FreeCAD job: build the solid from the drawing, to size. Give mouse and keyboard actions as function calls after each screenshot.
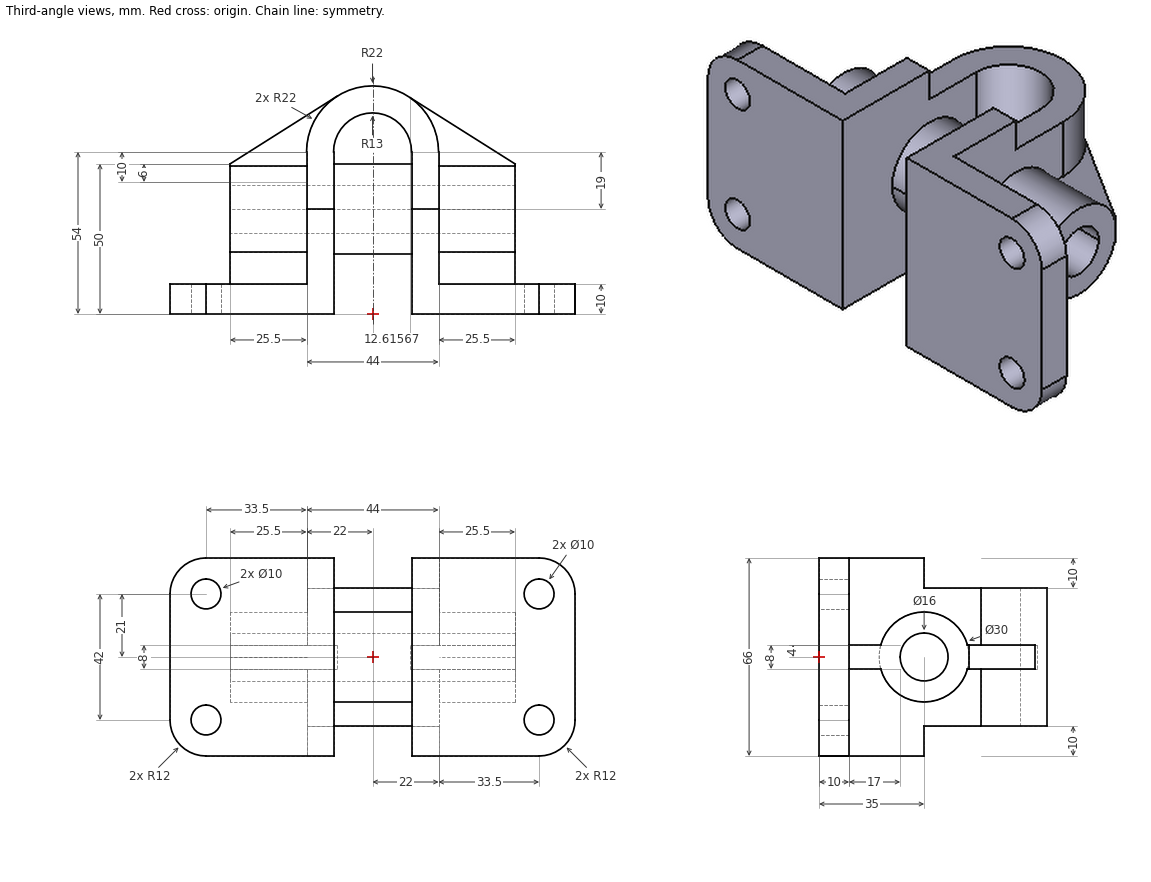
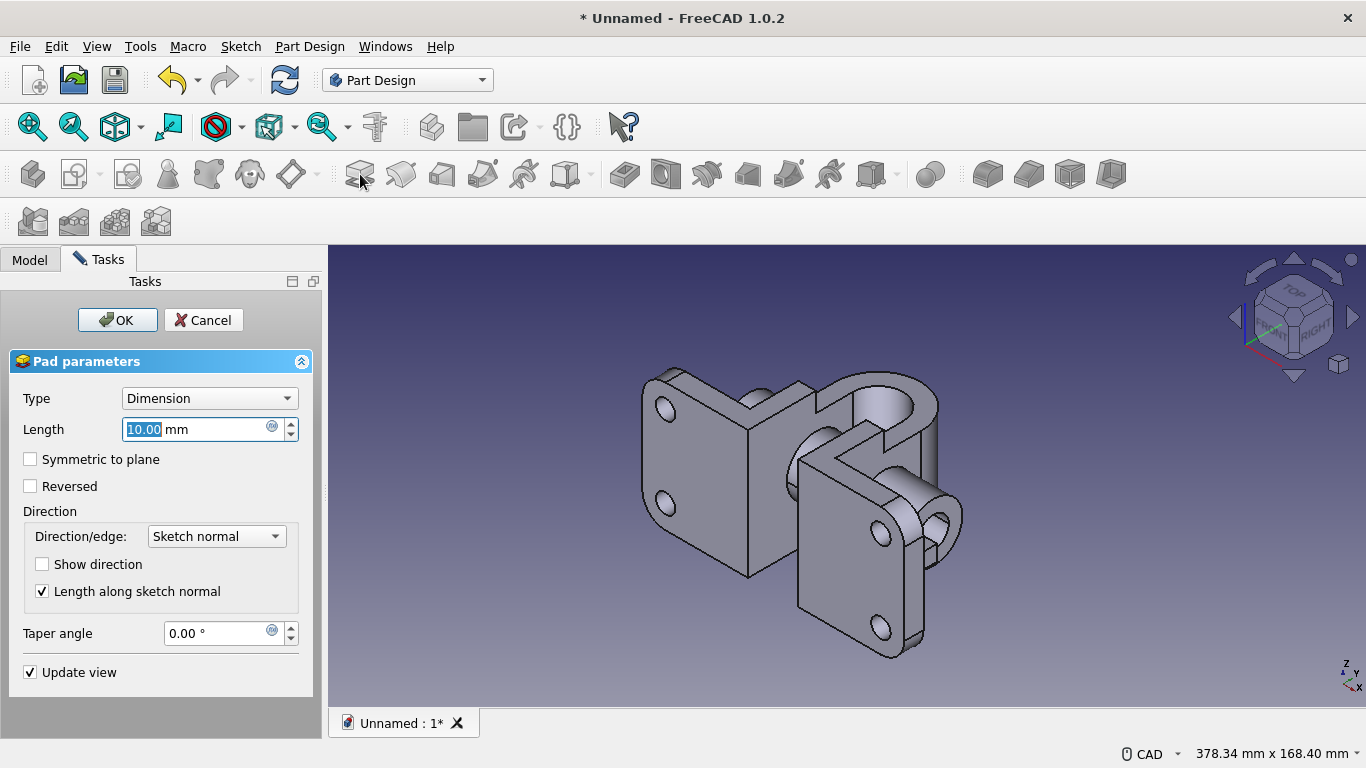
text(25.5)
key(Tab)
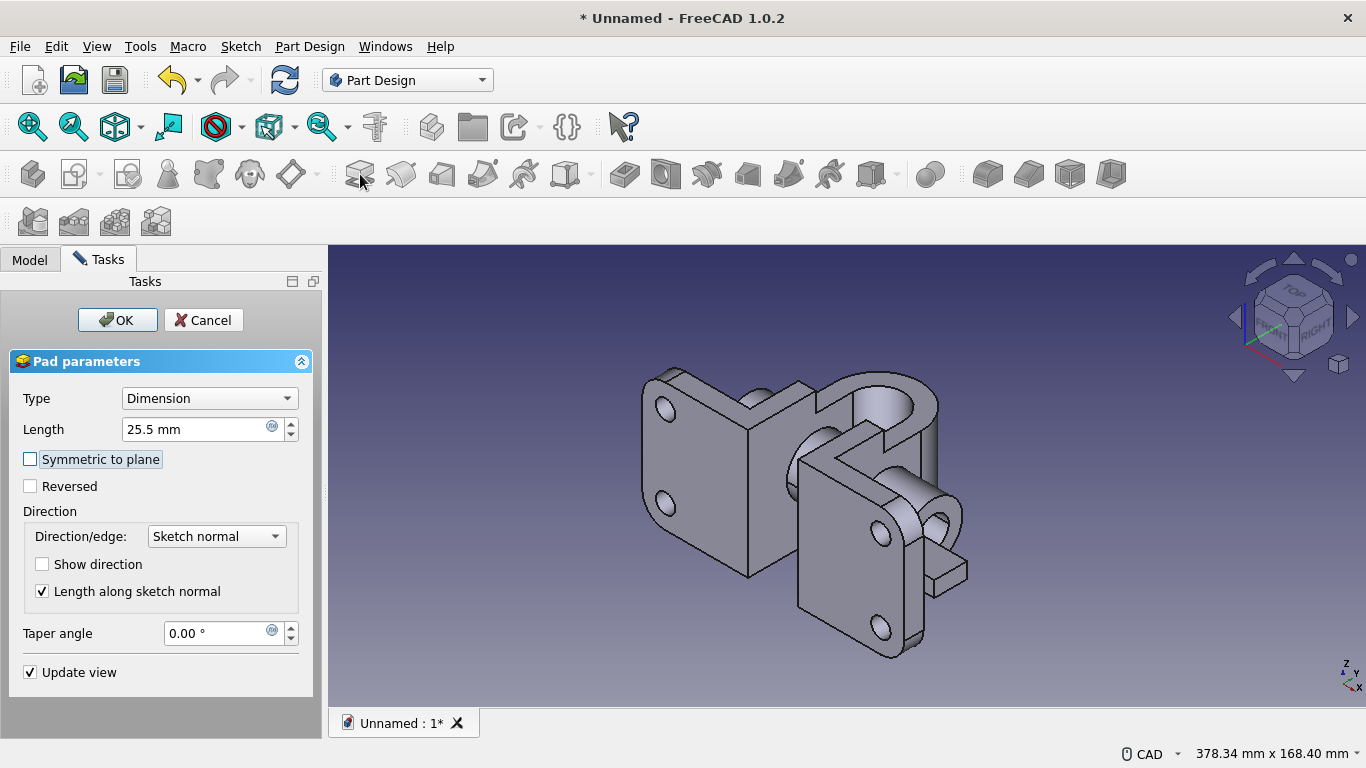
click(31, 486)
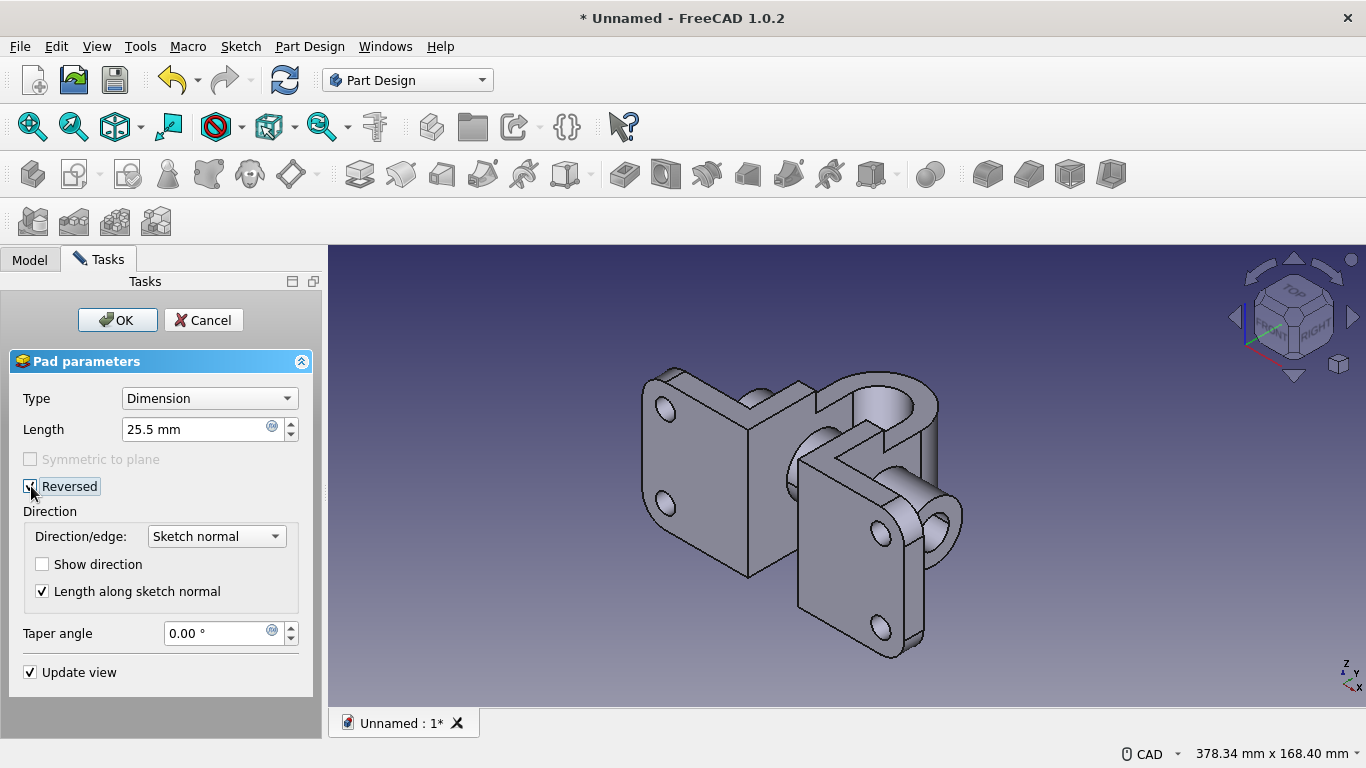
click(118, 320)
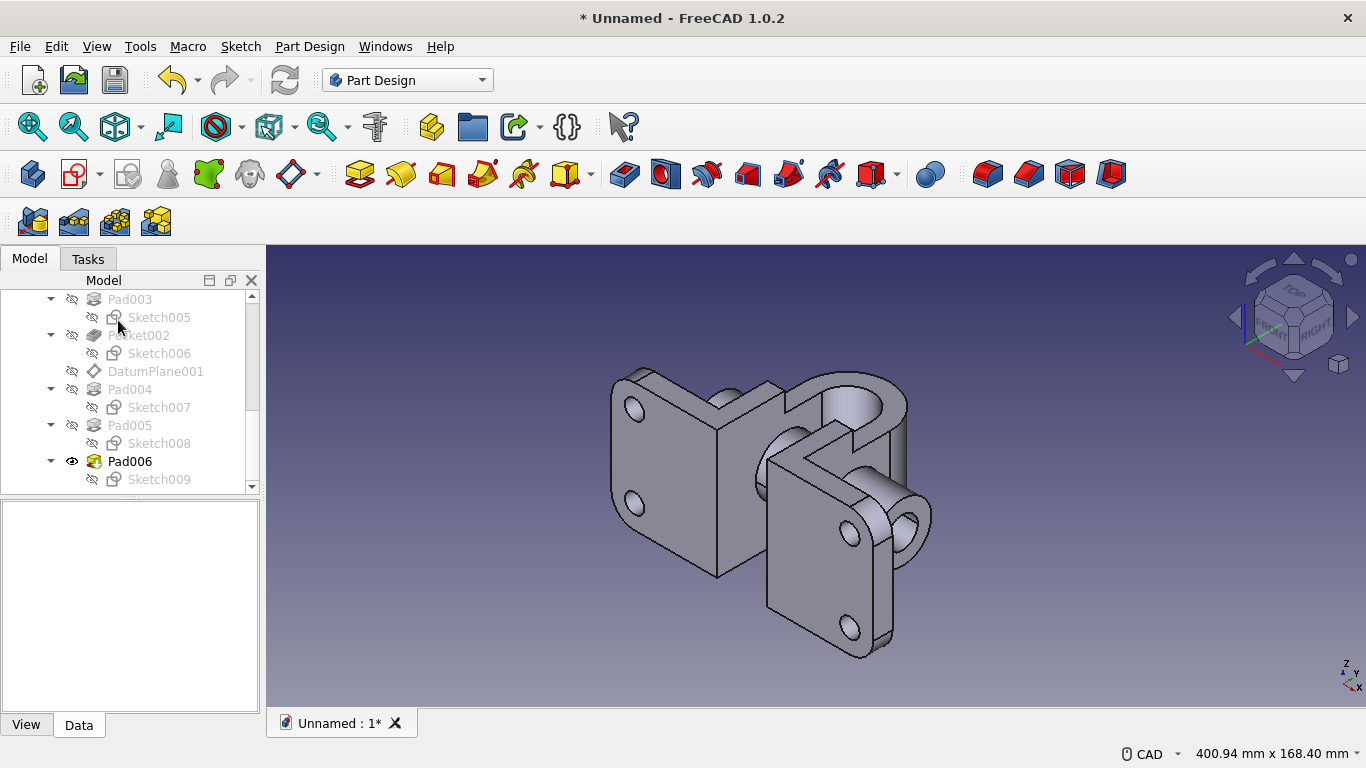
key(6)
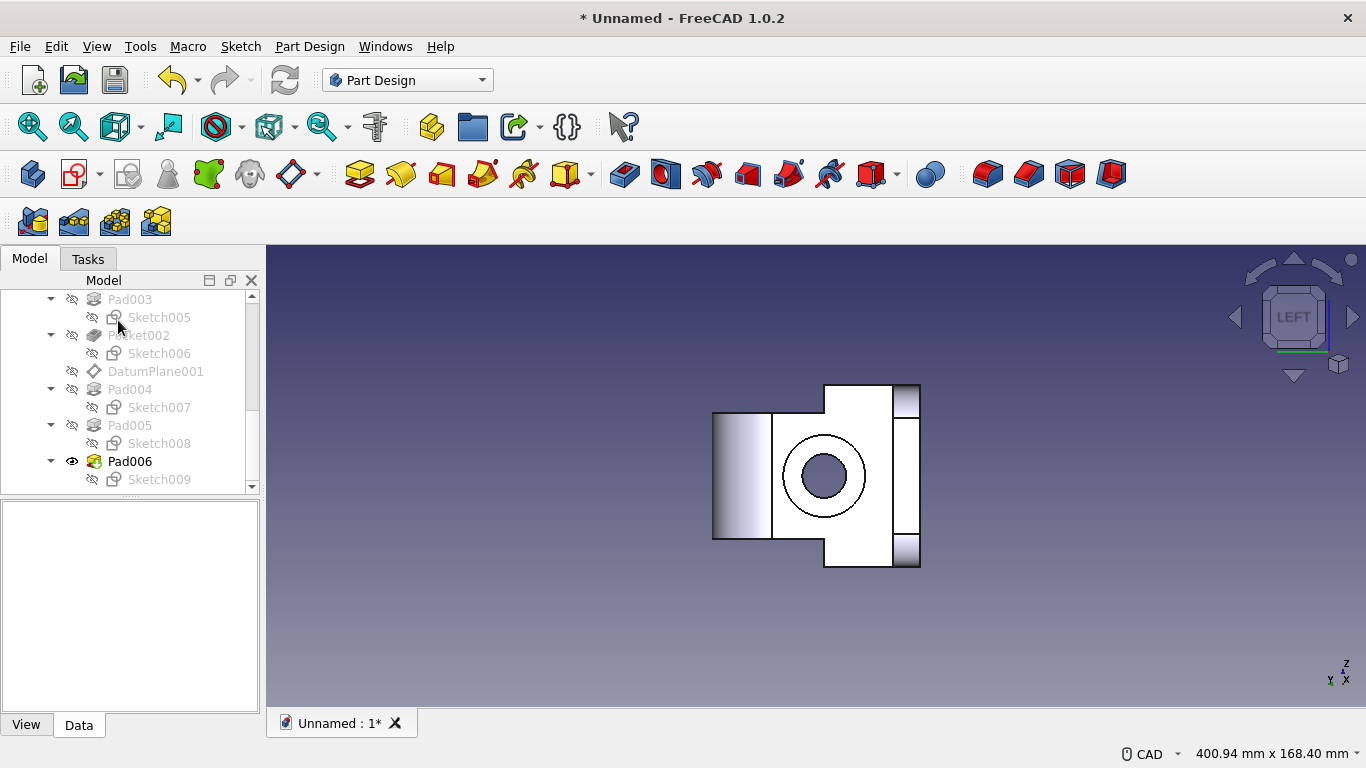
click(33, 128)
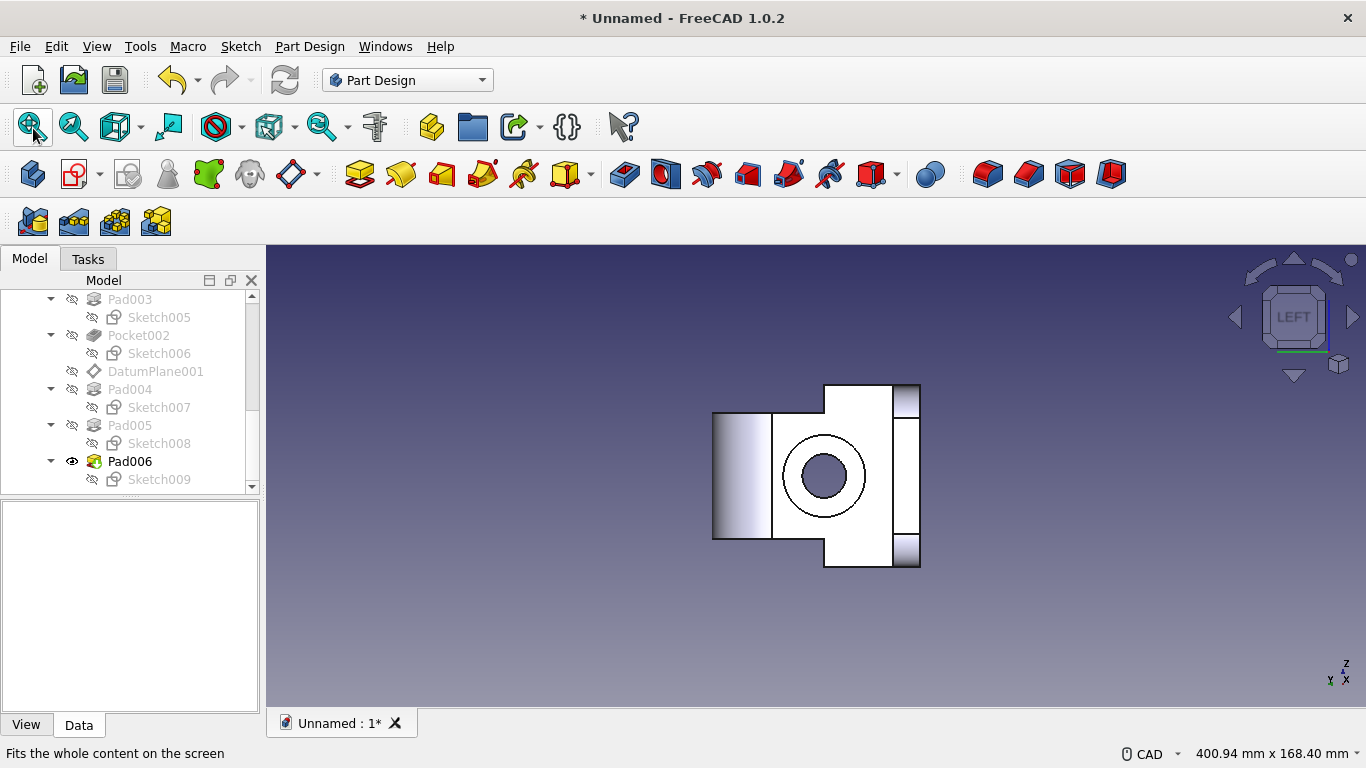
key(2)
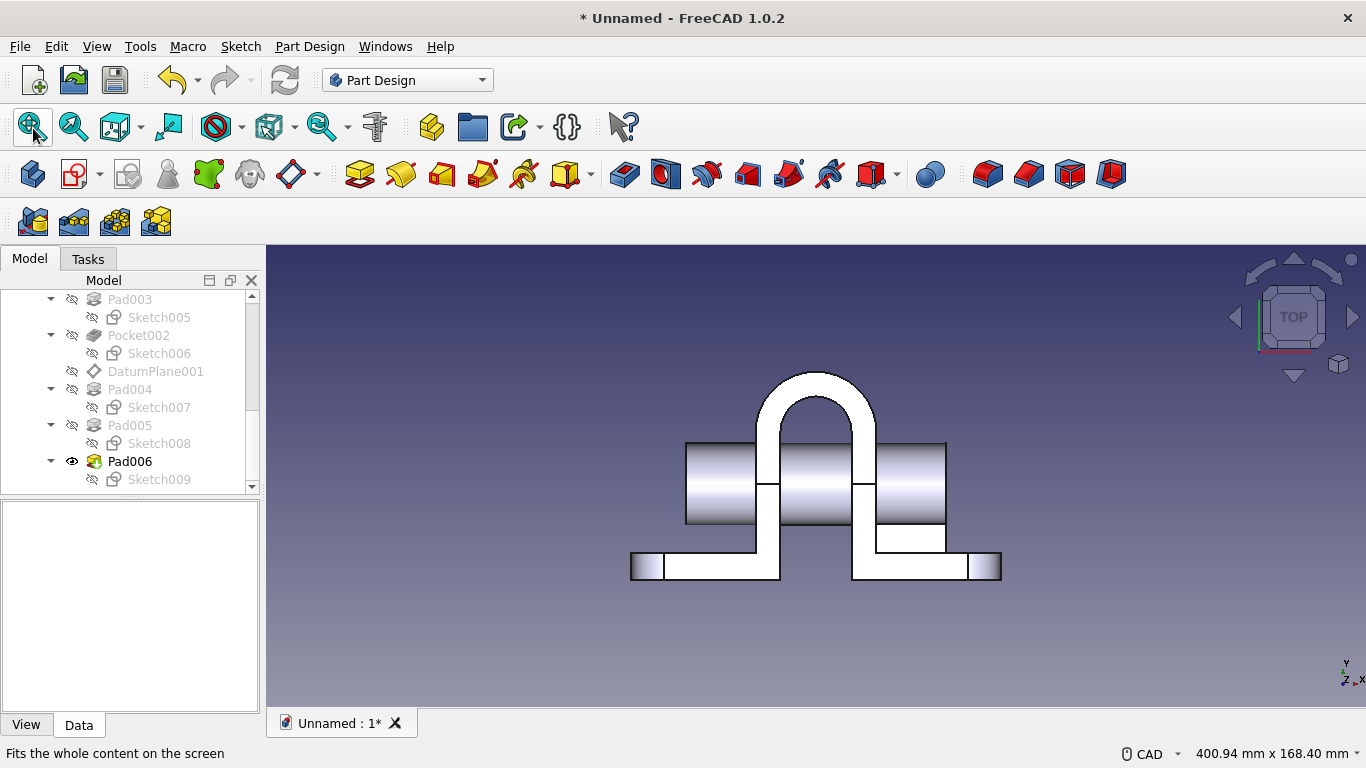
key(1)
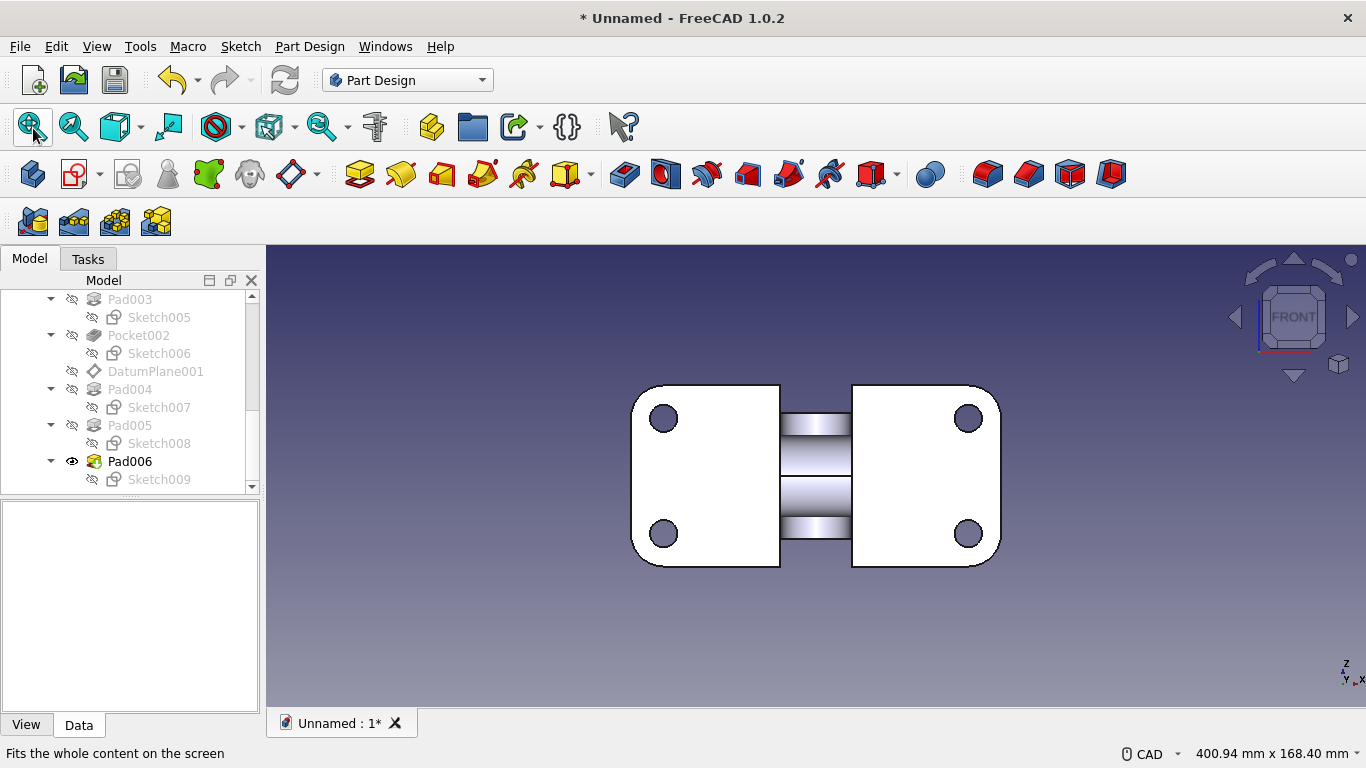
click(33, 128)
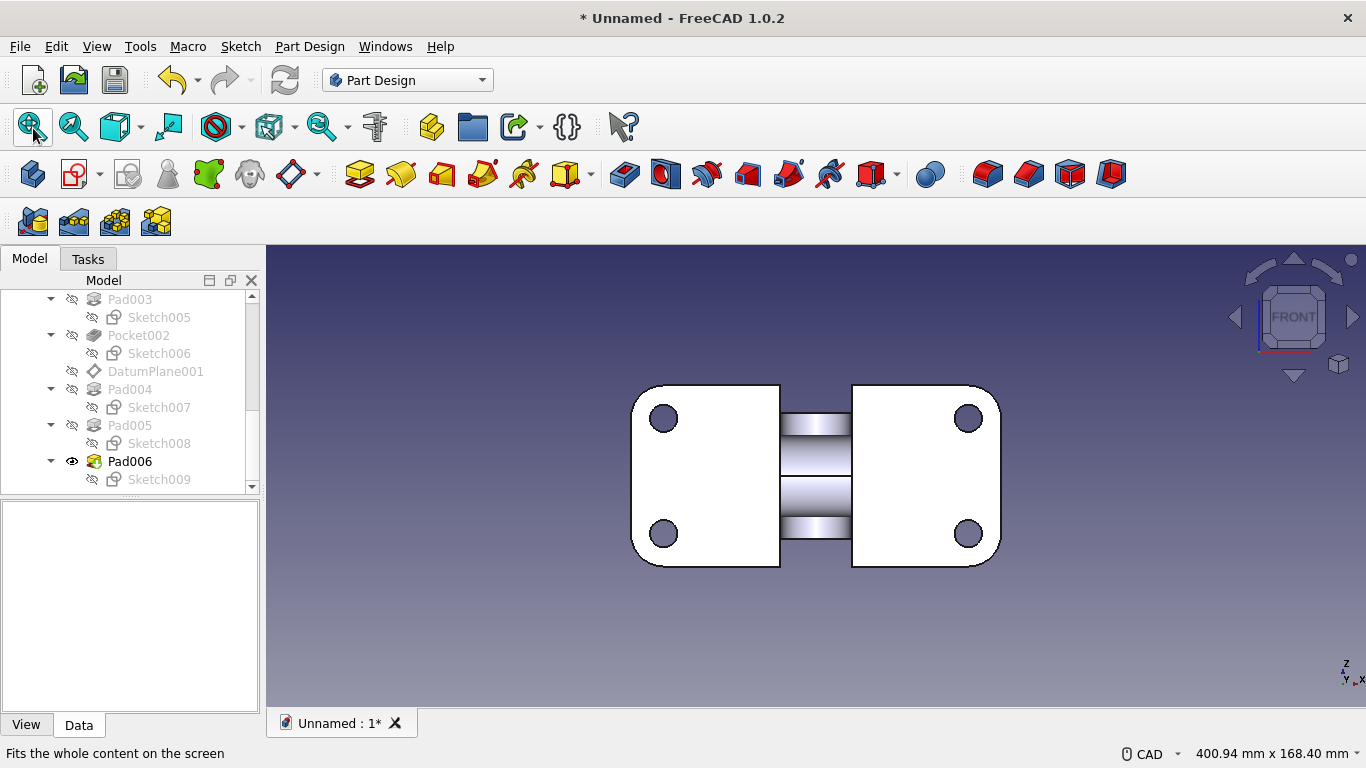
scroll(141, 385, down, 3)